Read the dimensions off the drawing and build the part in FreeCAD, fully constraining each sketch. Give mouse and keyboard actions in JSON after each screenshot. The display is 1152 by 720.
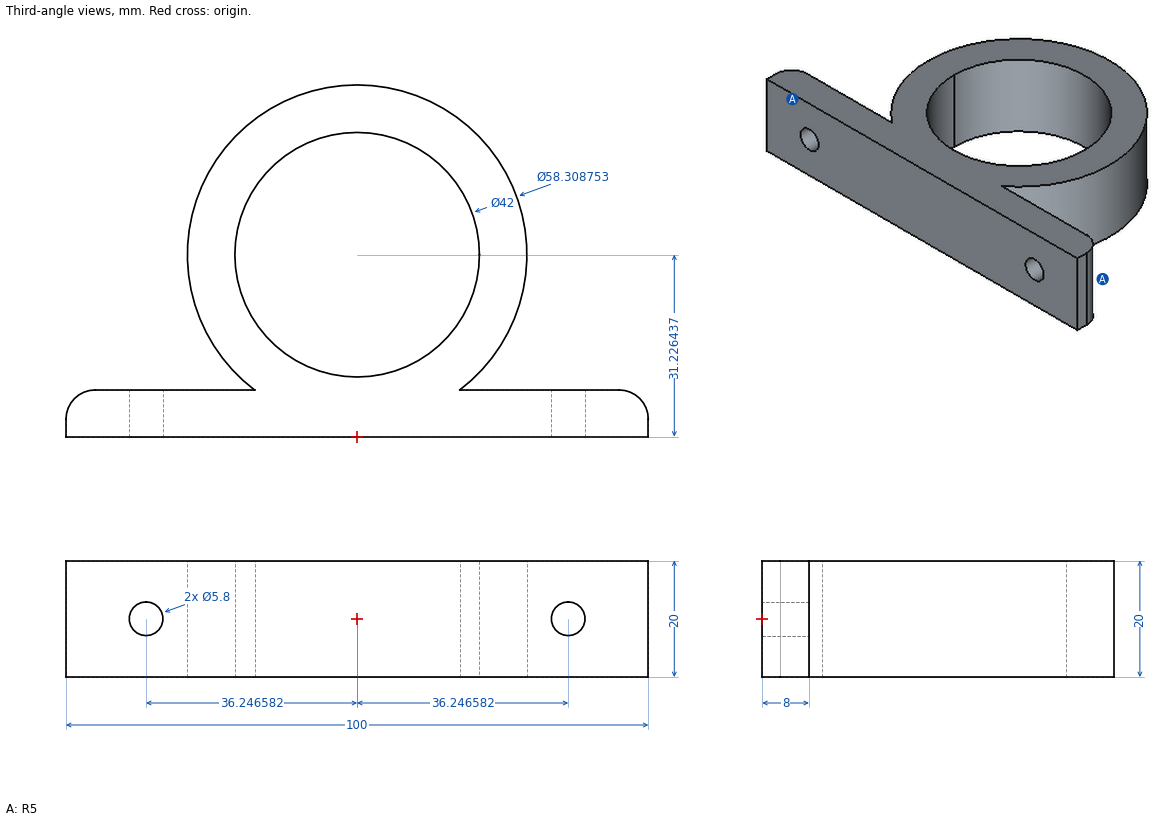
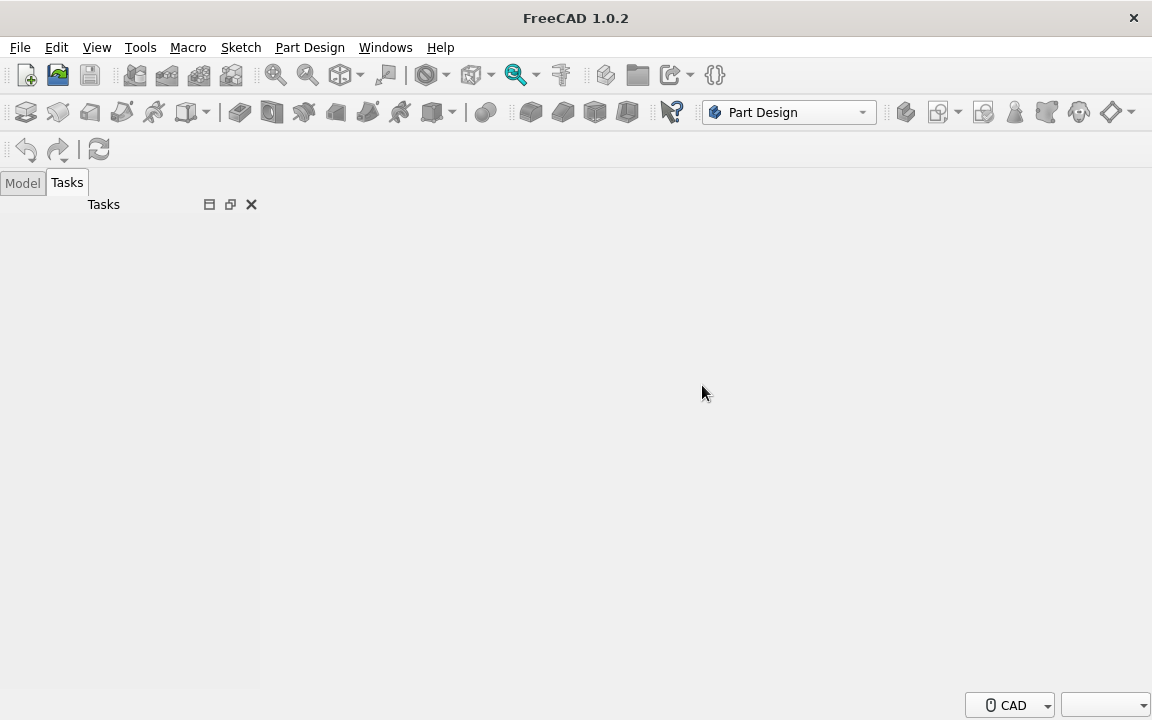
{"action": "left_click", "coordinate": [26, 76]}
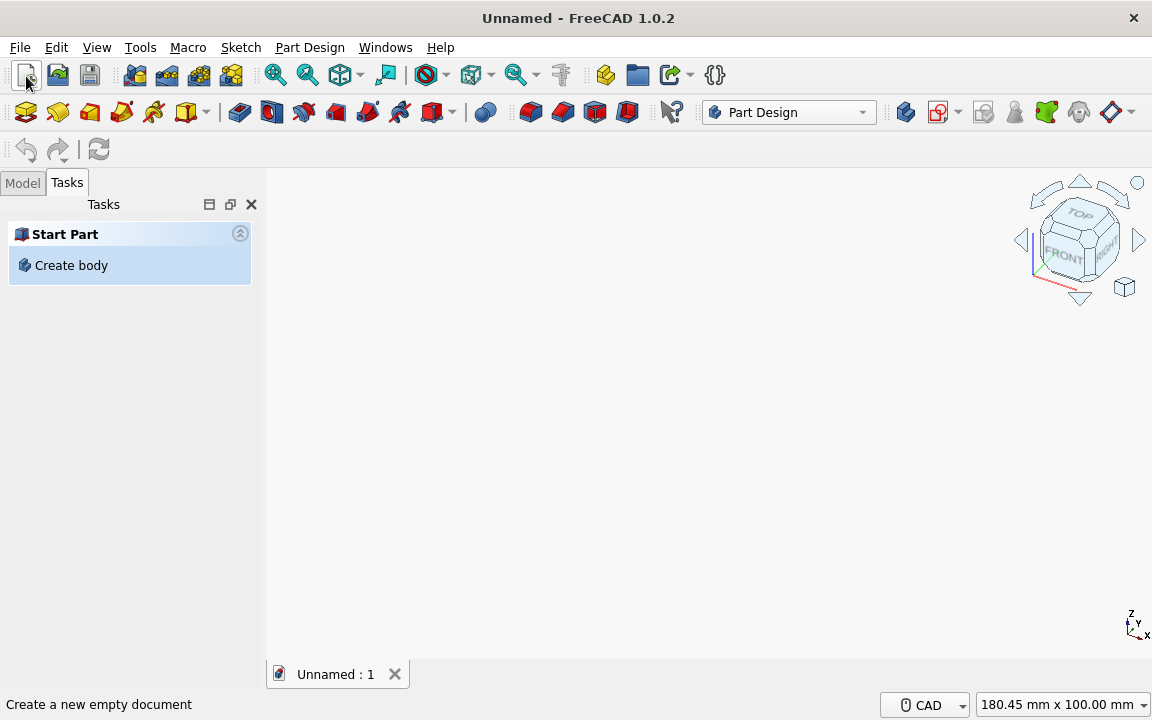
{"action": "left_click", "coordinate": [938, 112]}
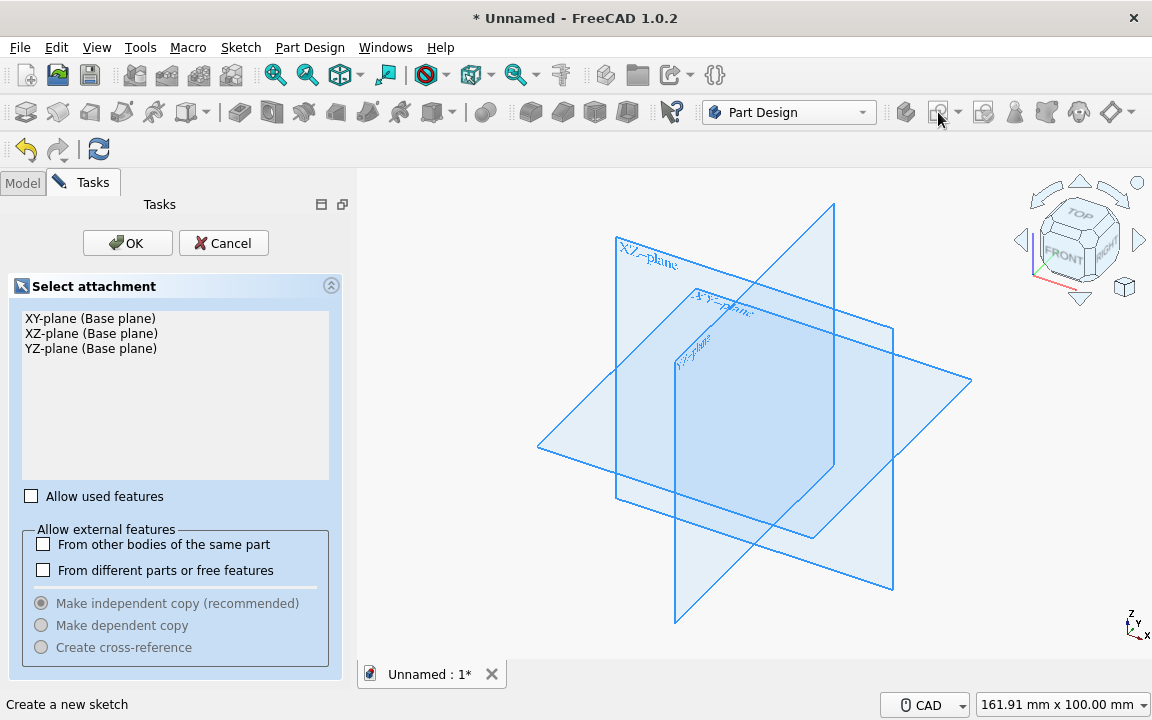
{"action": "left_click", "coordinate": [82, 334]}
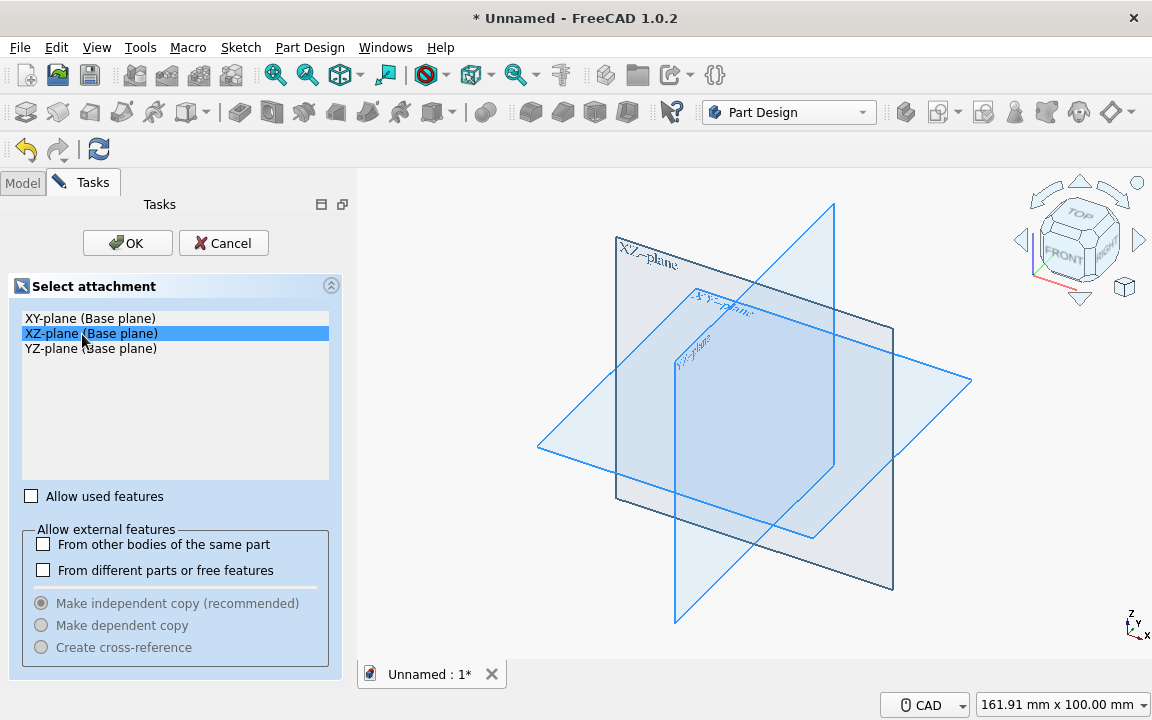
{"action": "left_click", "coordinate": [128, 243]}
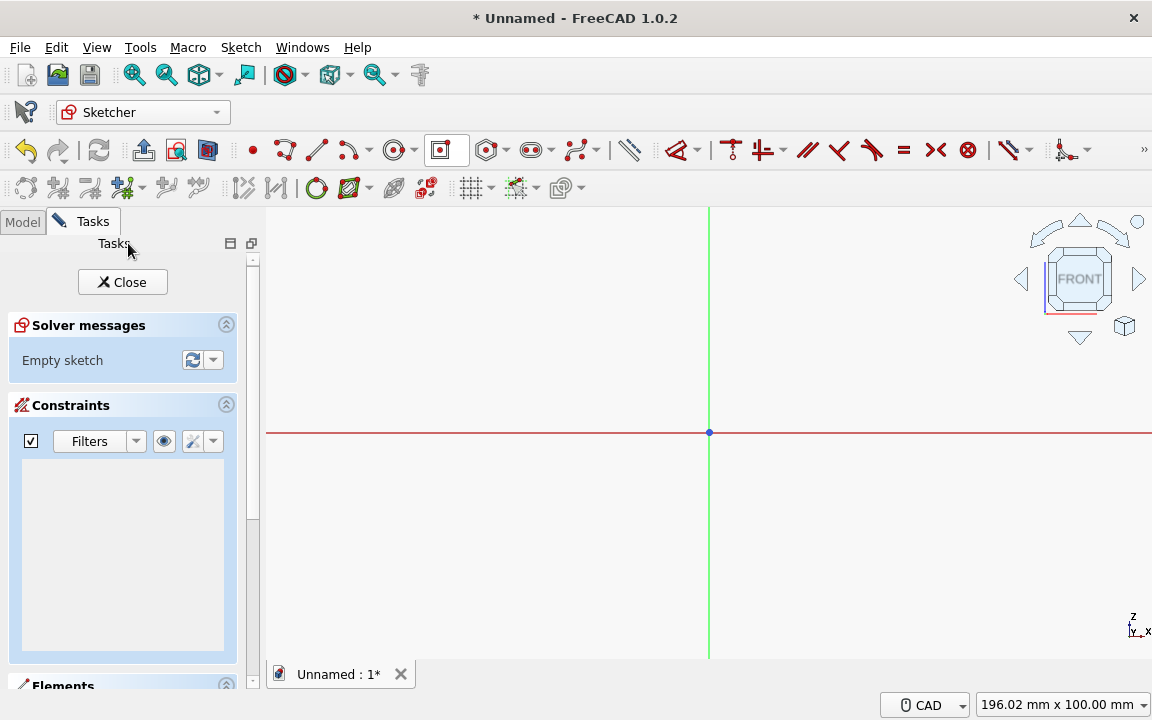
{"action": "left_click", "coordinate": [440, 150]}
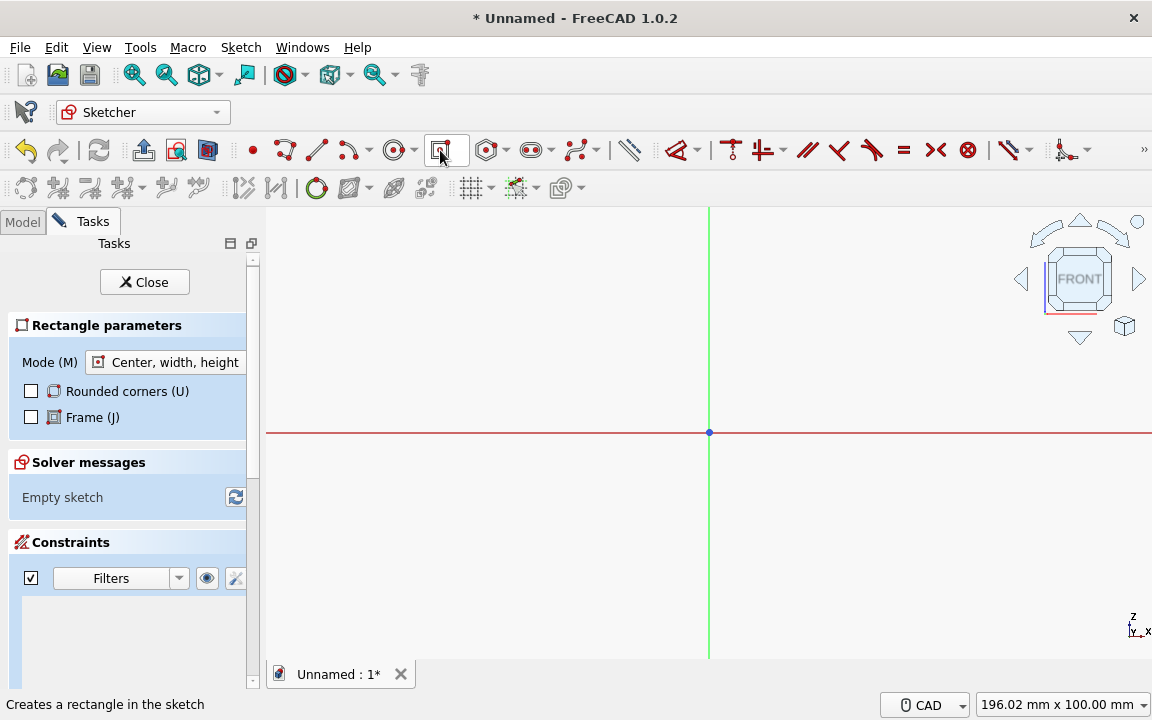
{"action": "left_click", "coordinate": [709, 433]}
{"action": "left_click", "coordinate": [935, 388]}
{"action": "key", "text": "Escape"}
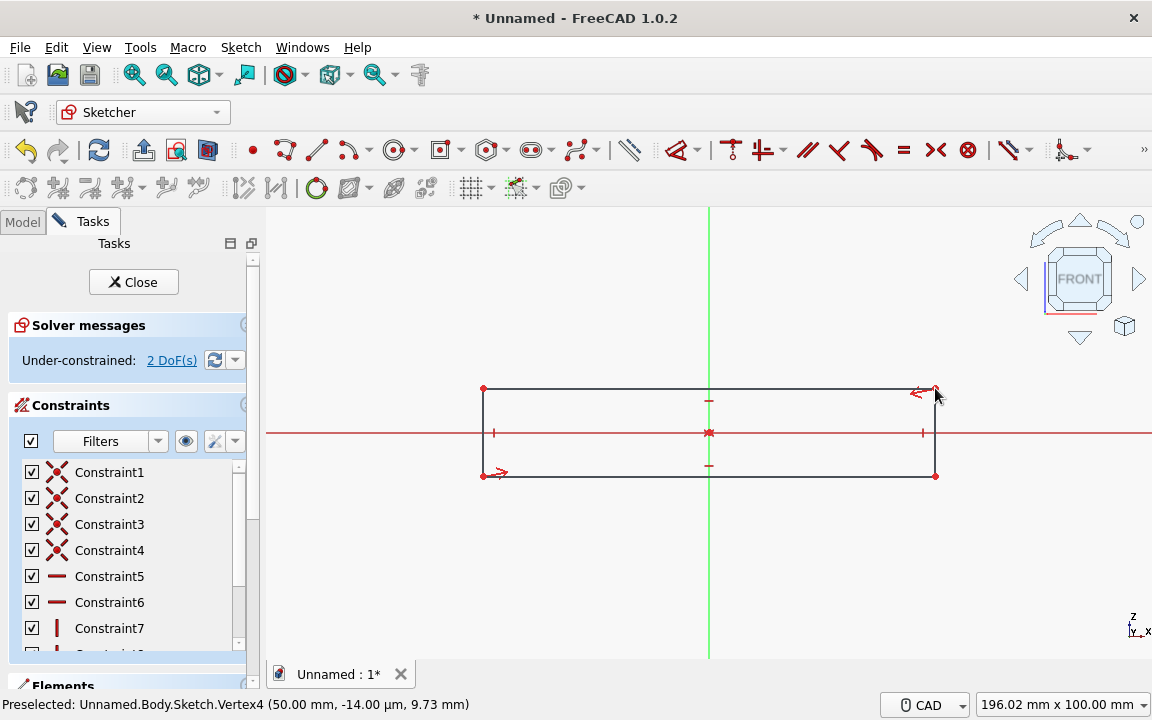
{"action": "left_click", "coordinate": [676, 150]}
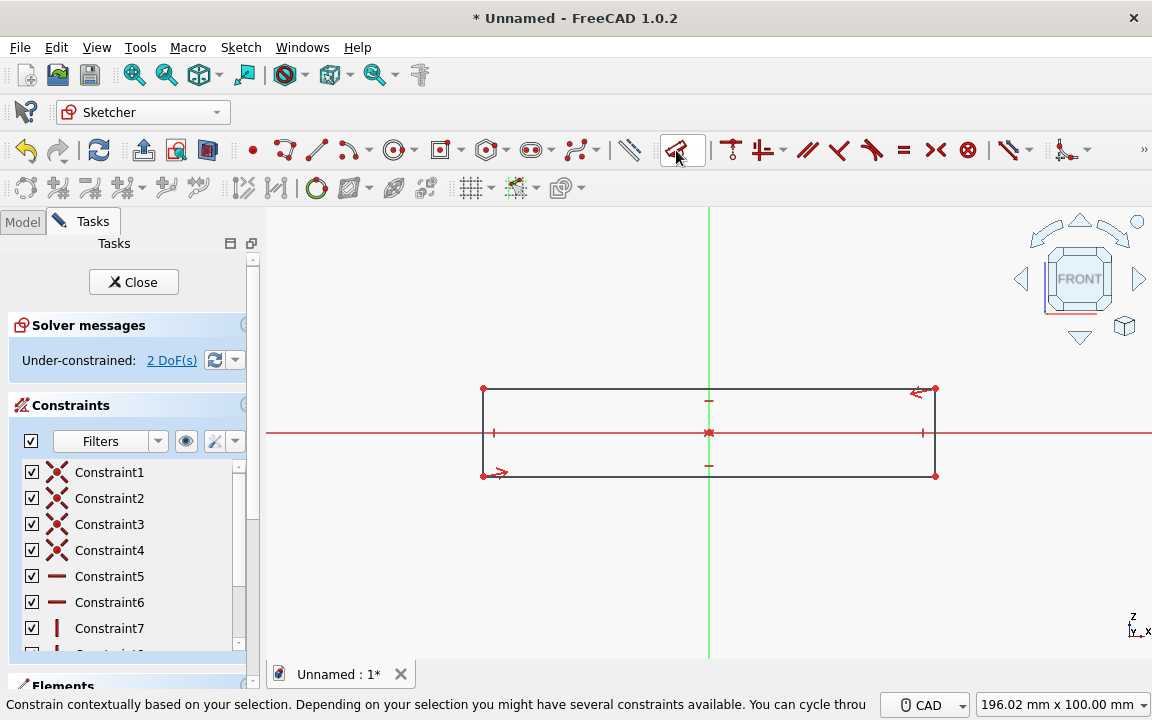
{"action": "left_click", "coordinate": [935, 451]}
{"action": "left_click", "coordinate": [969, 413]}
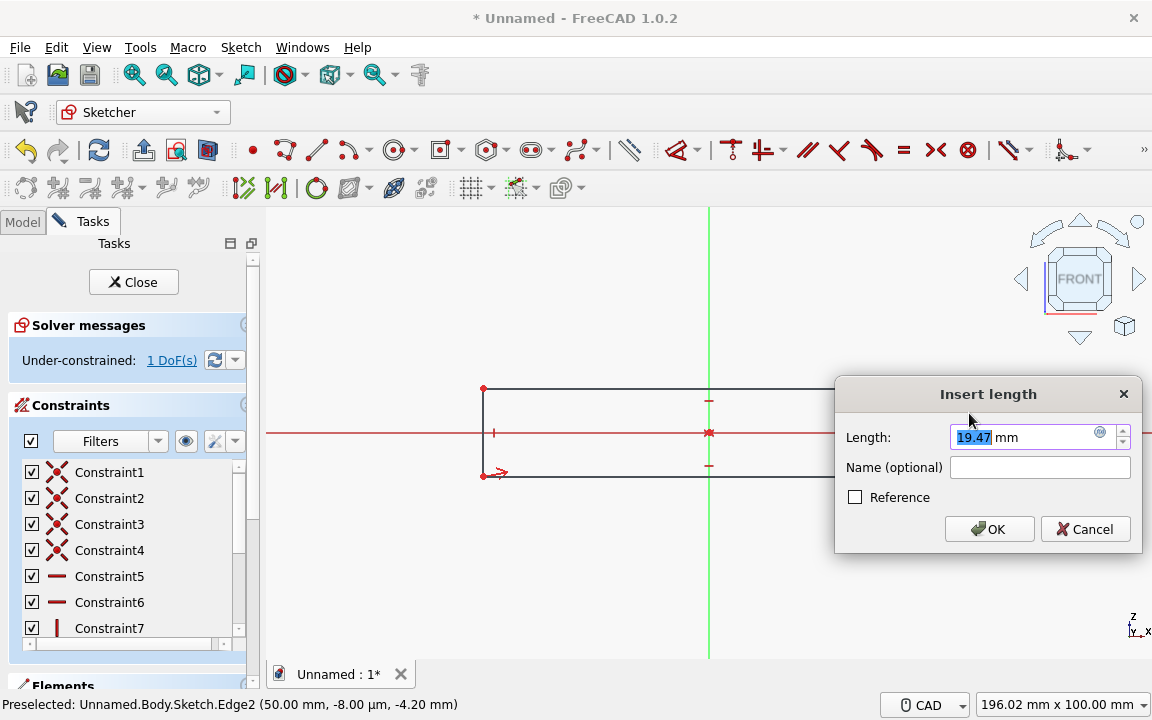
{"action": "type", "text": "20"}
{"action": "key", "text": "Return"}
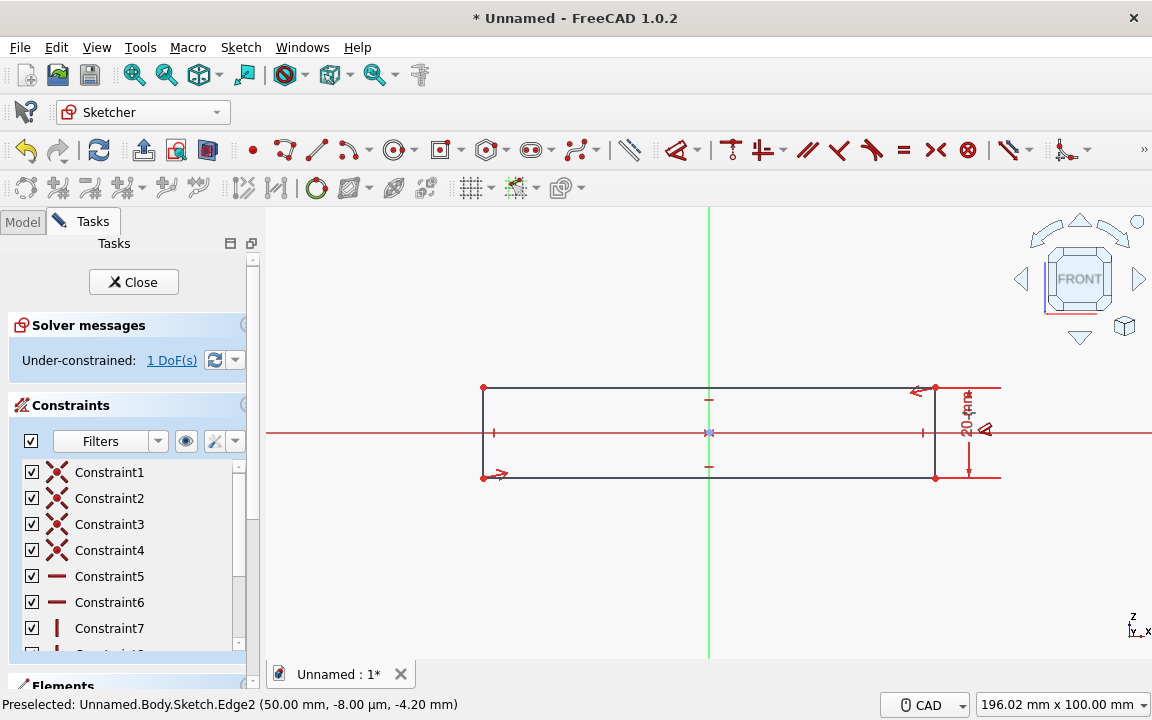
{"action": "left_click", "coordinate": [619, 478]}
{"action": "left_click", "coordinate": [605, 512]}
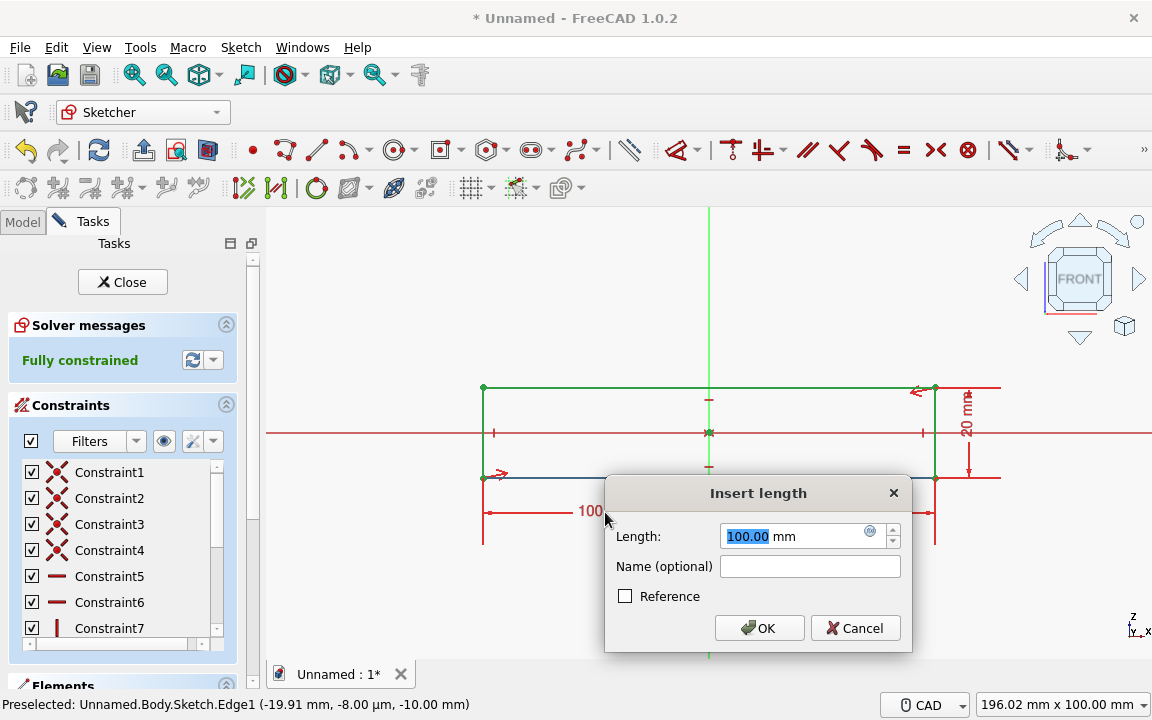
{"action": "type", "text": "100"}
{"action": "key", "text": "Return"}
{"action": "key", "text": "Escape"}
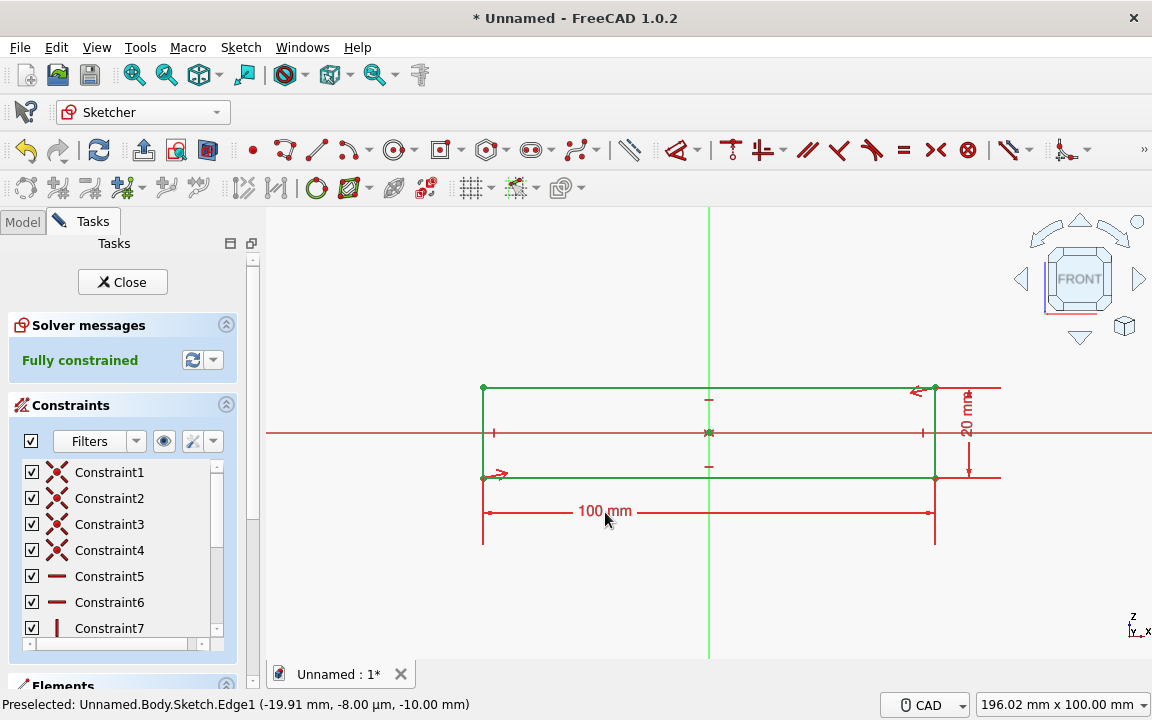
{"action": "left_click", "coordinate": [123, 282]}